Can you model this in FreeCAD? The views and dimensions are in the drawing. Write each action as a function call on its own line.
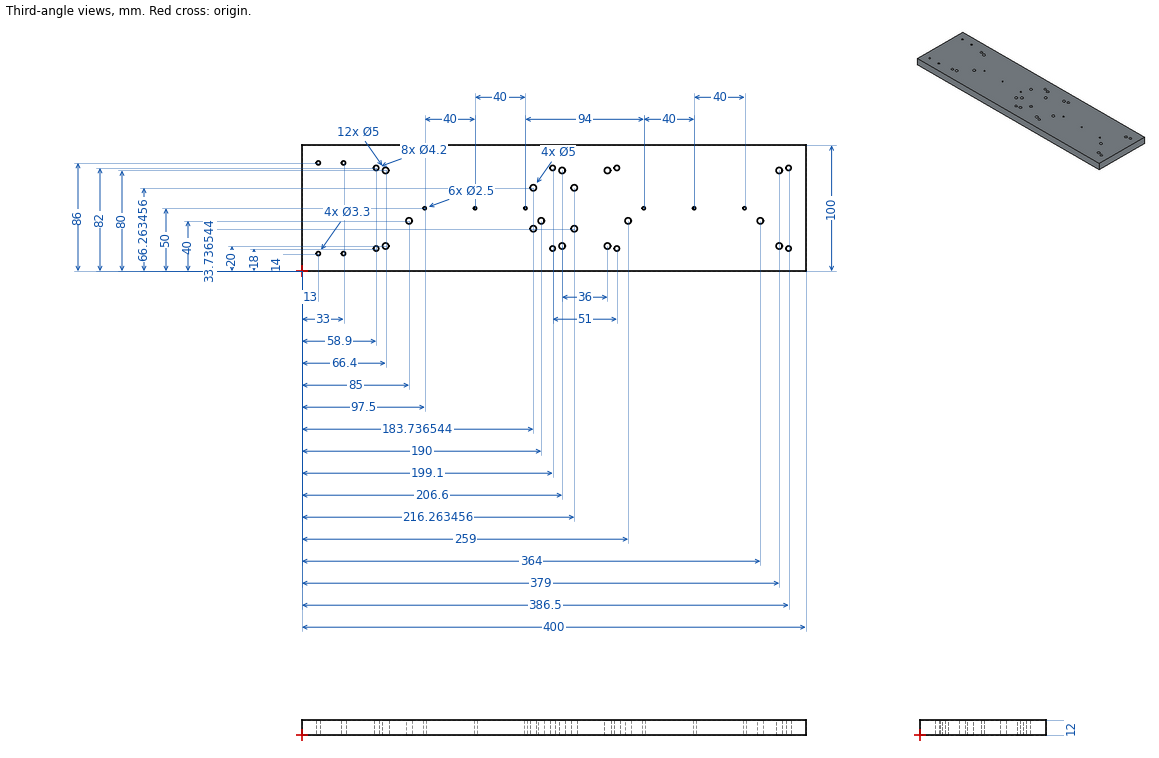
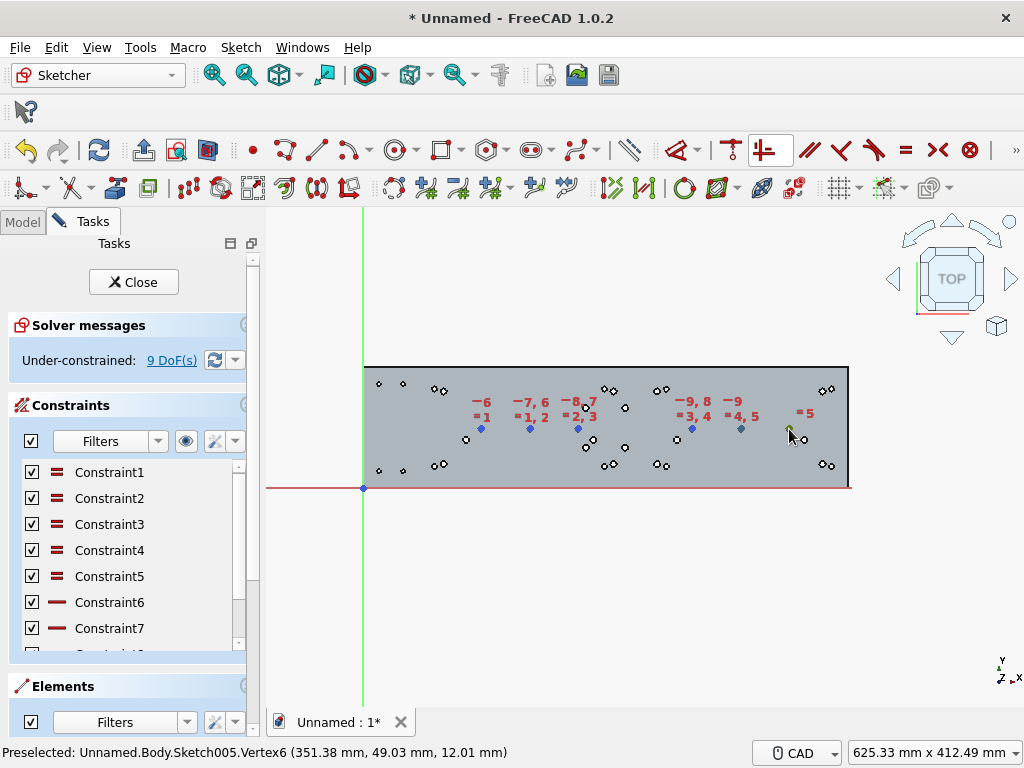
key(h)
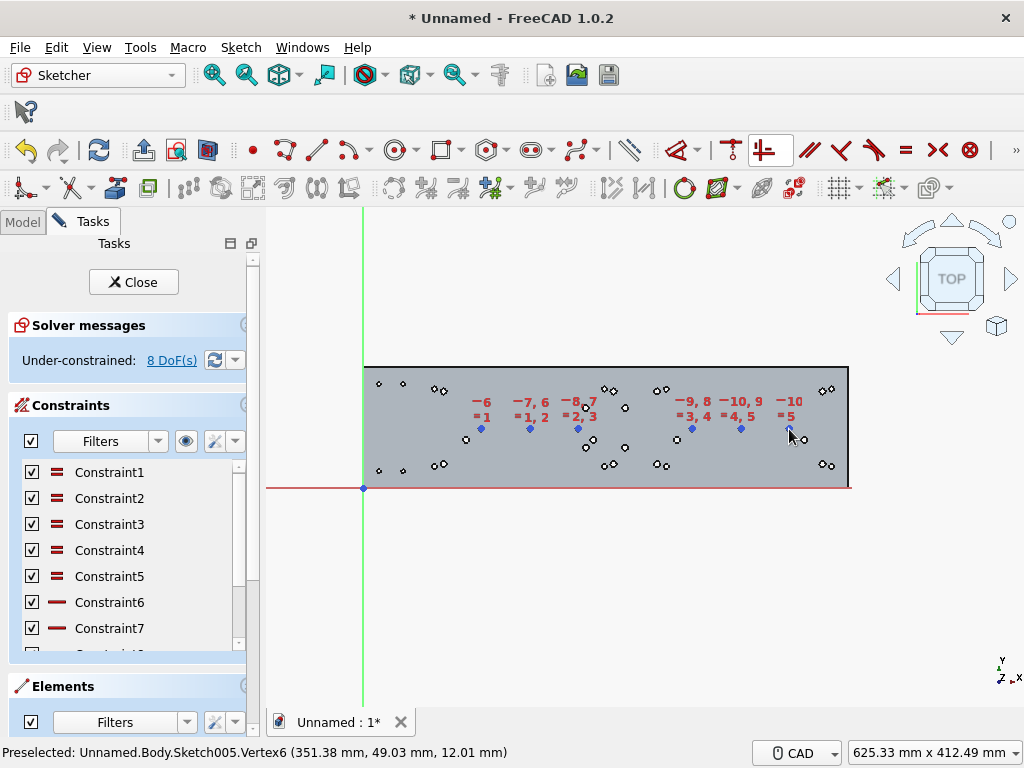
click(676, 150)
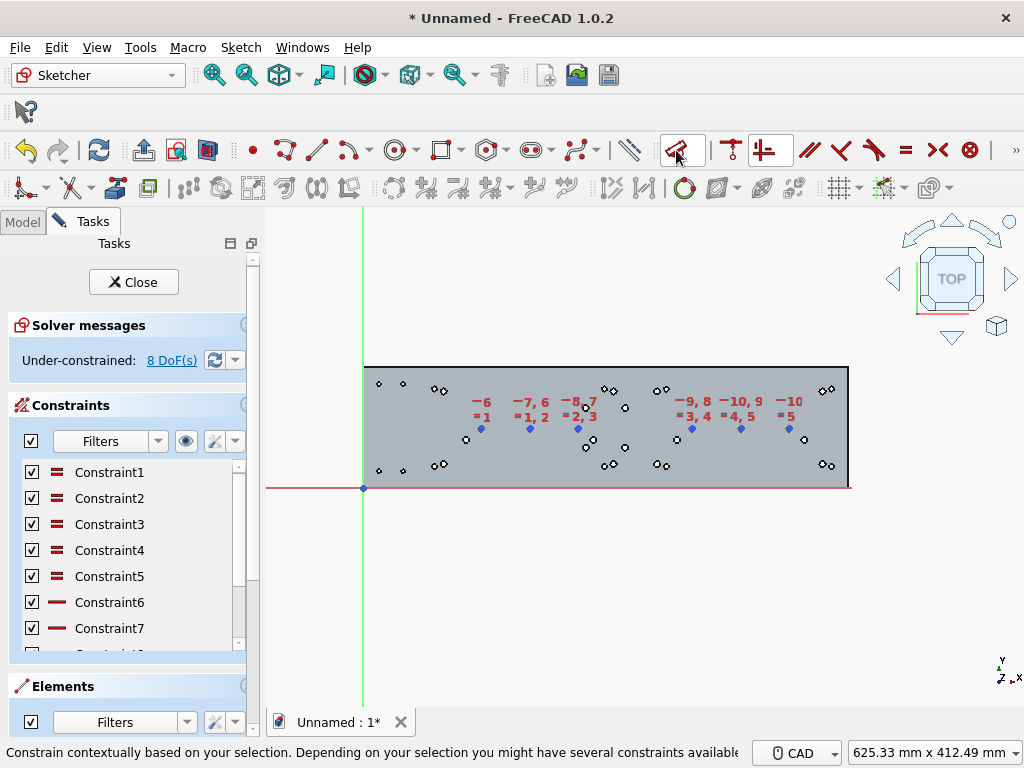
scroll(478, 429, up, 13)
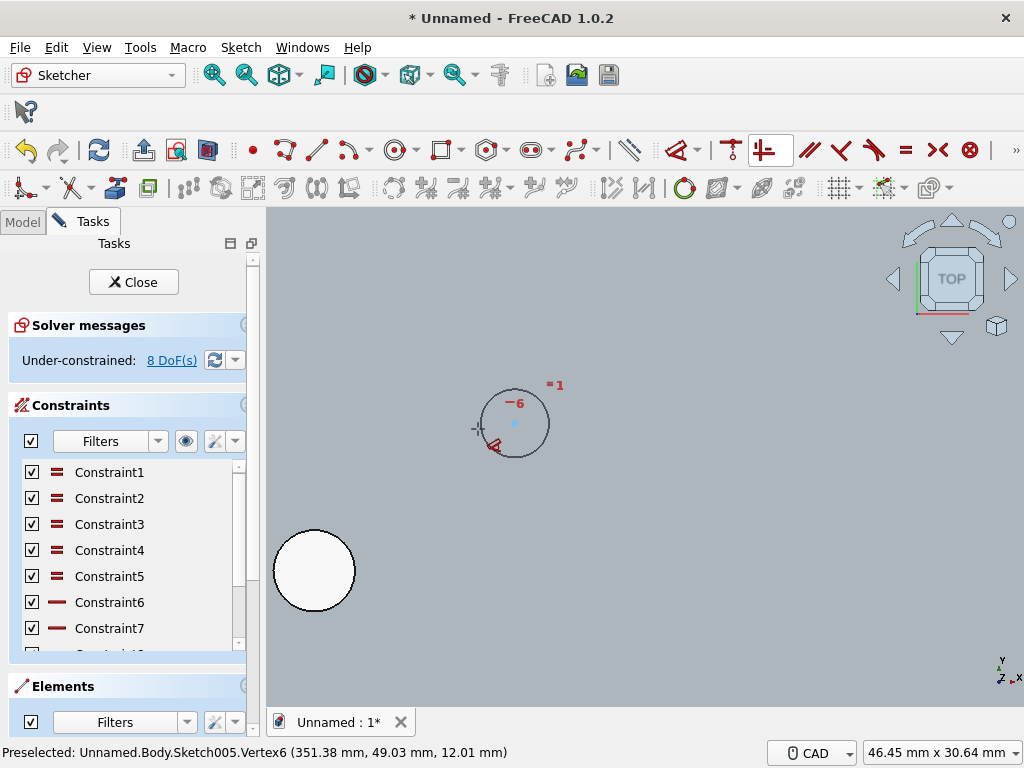
click(481, 422)
click(449, 421)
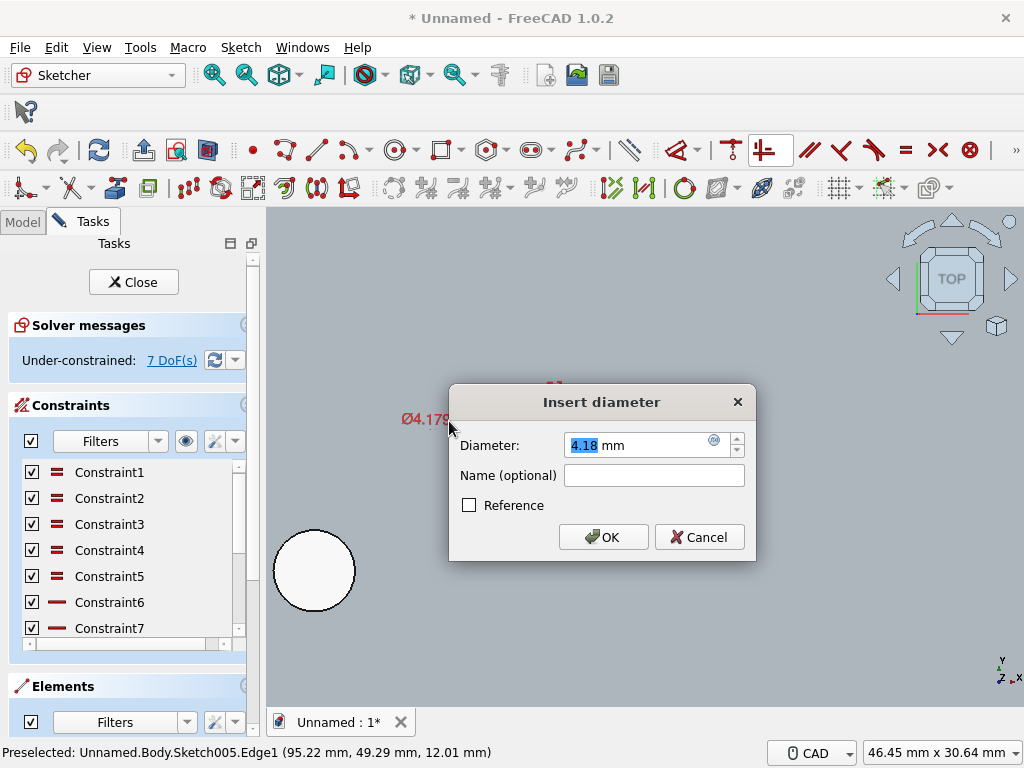
text(2.5)
key(Return)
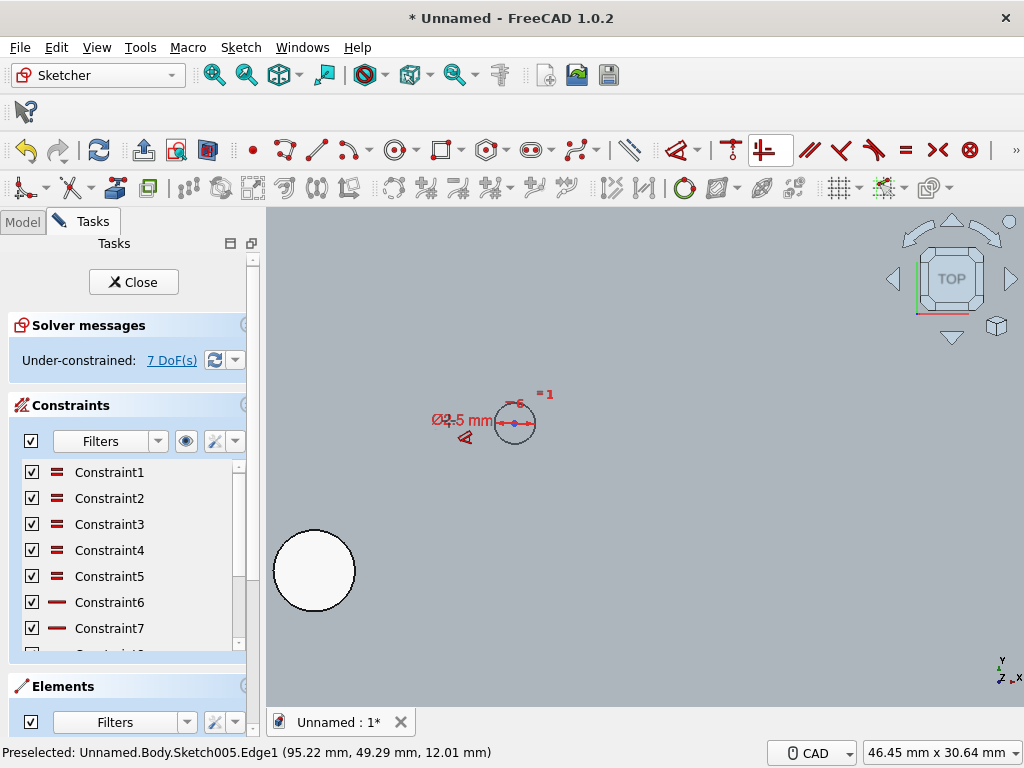
scroll(478, 429, down, 13)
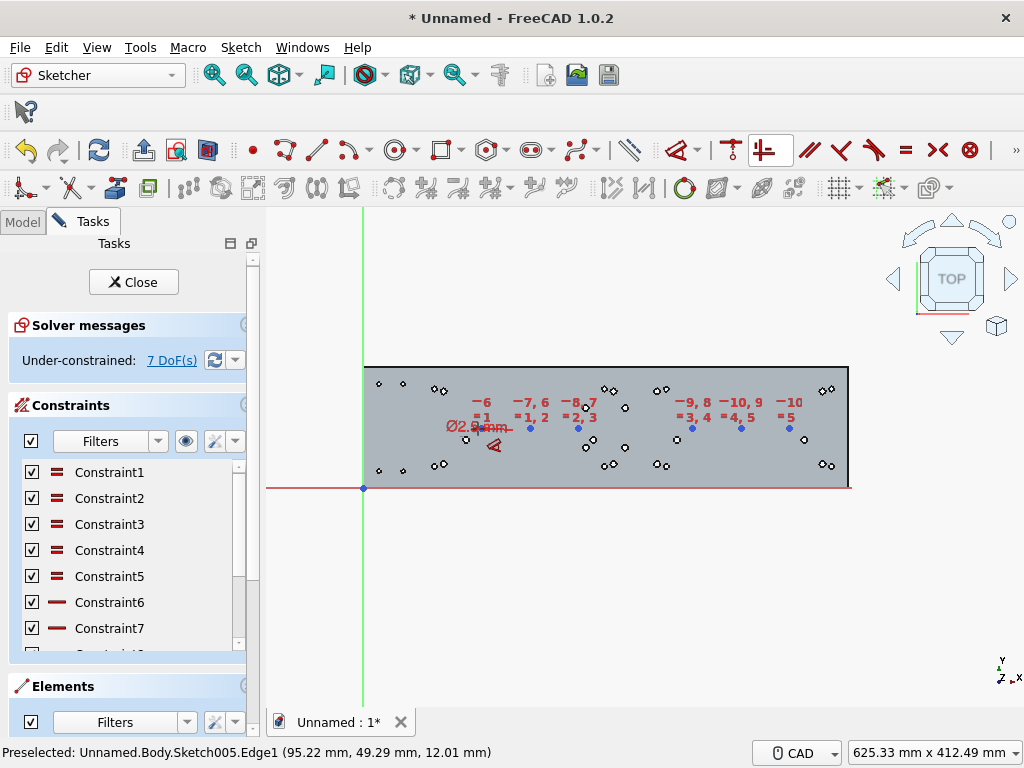
click(481, 429)
click(329, 459)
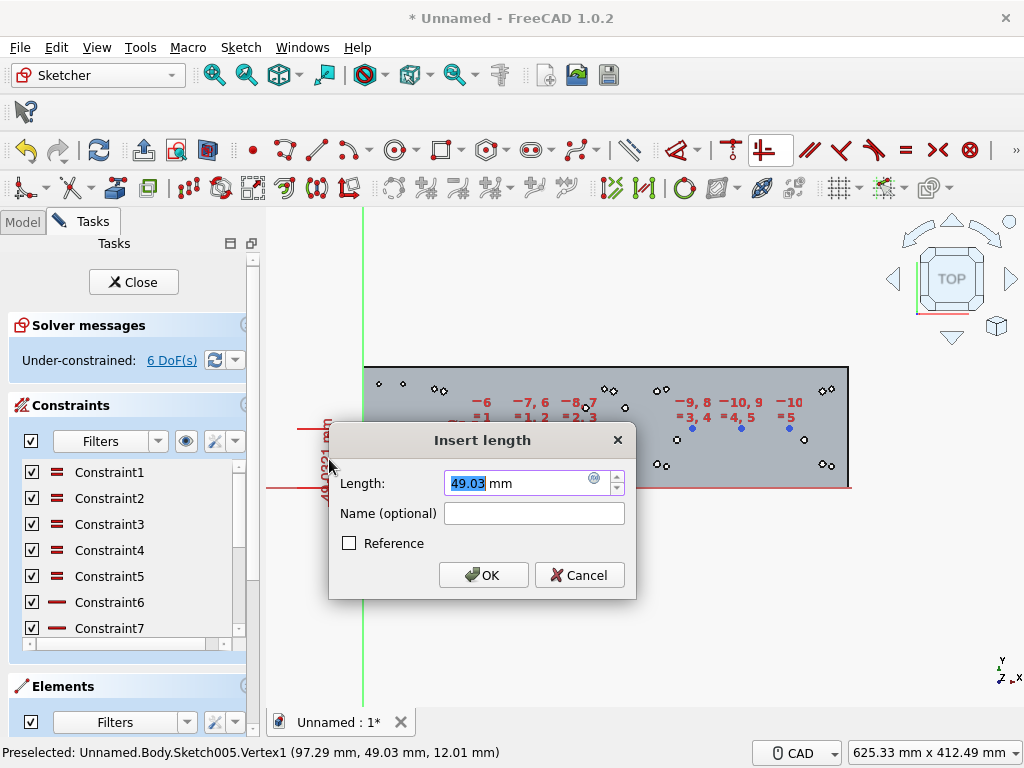
text(50)
key(Return)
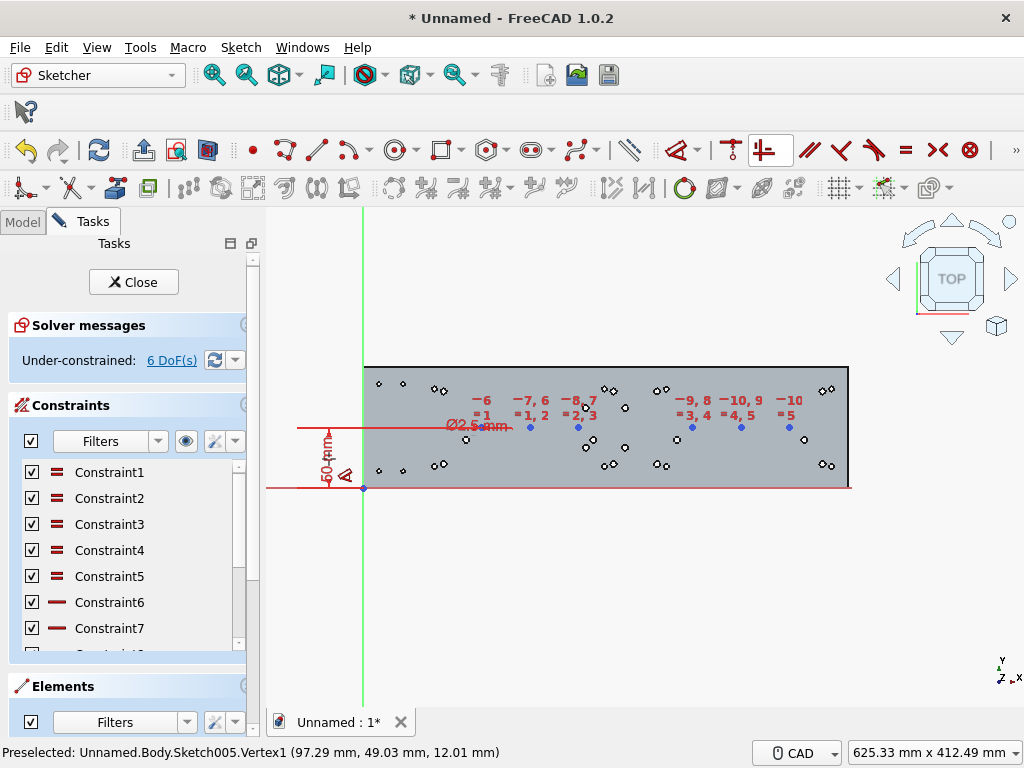
click(481, 428)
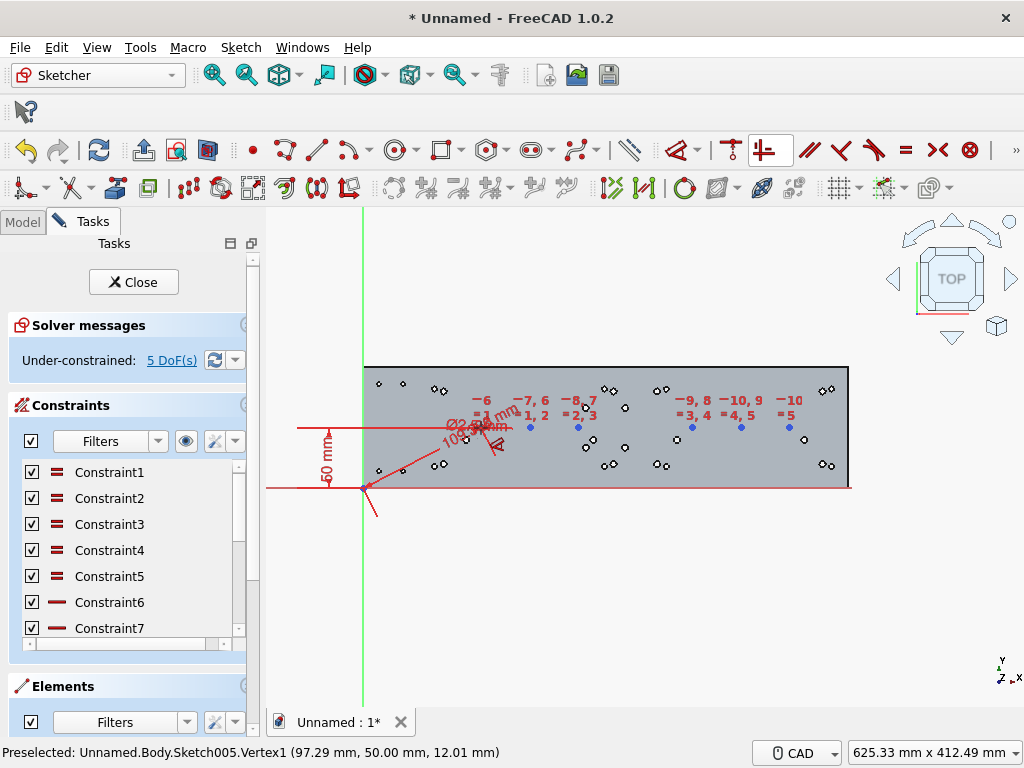
click(530, 428)
click(506, 394)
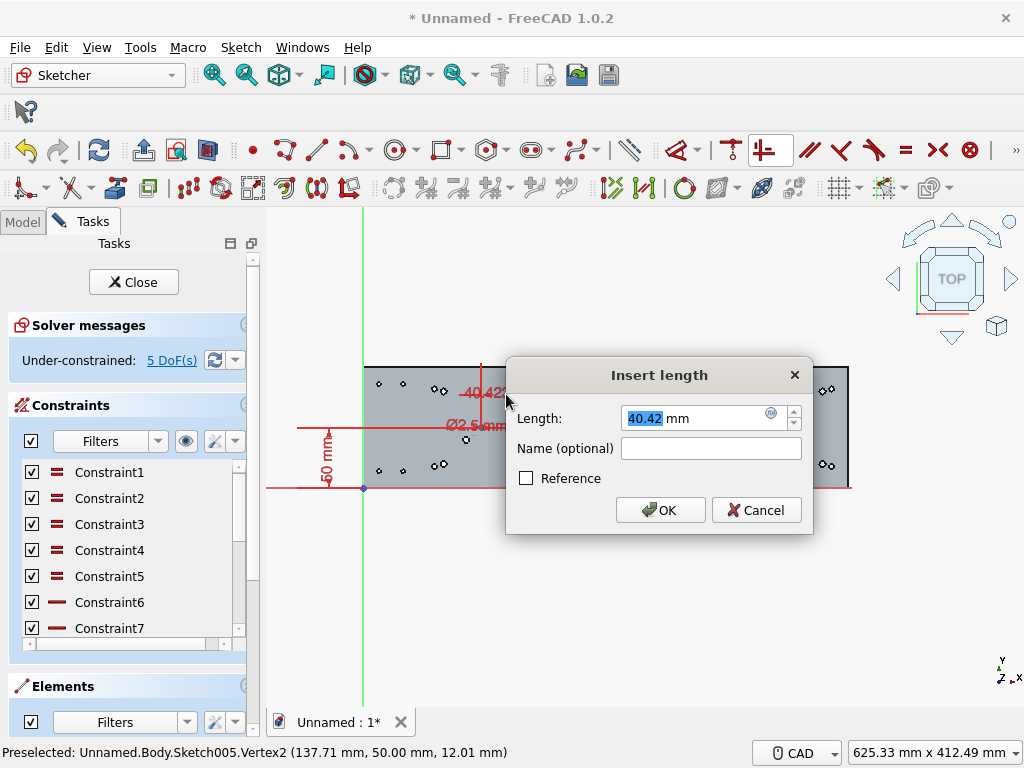
text(40)
key(Return)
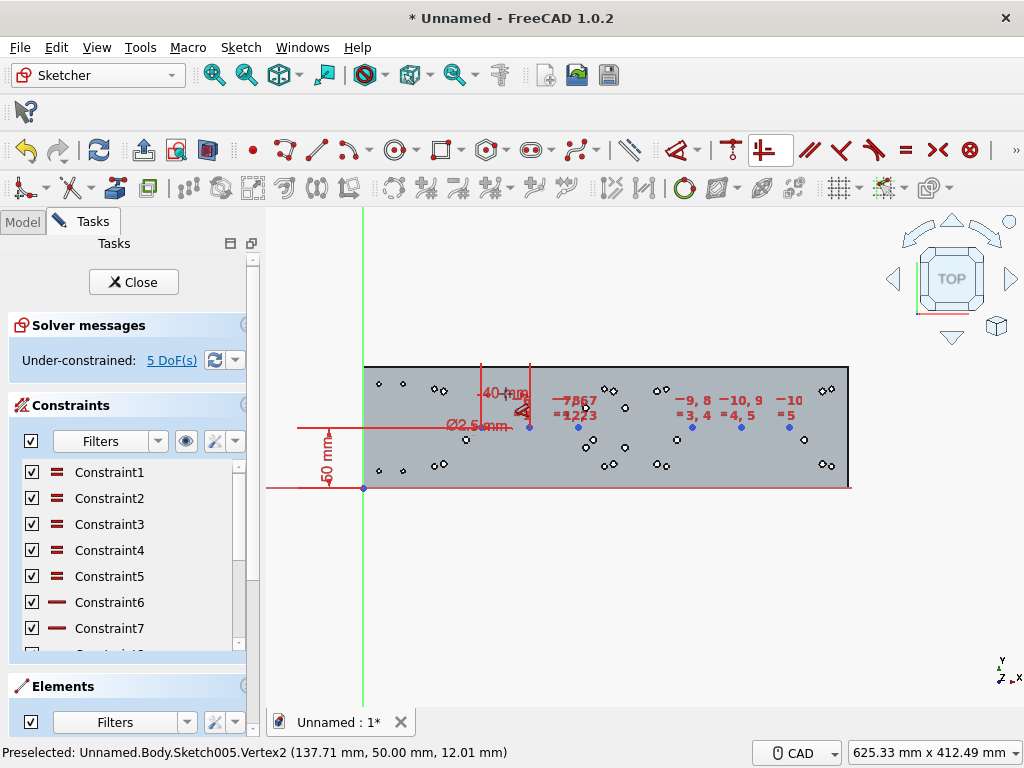
click(530, 428)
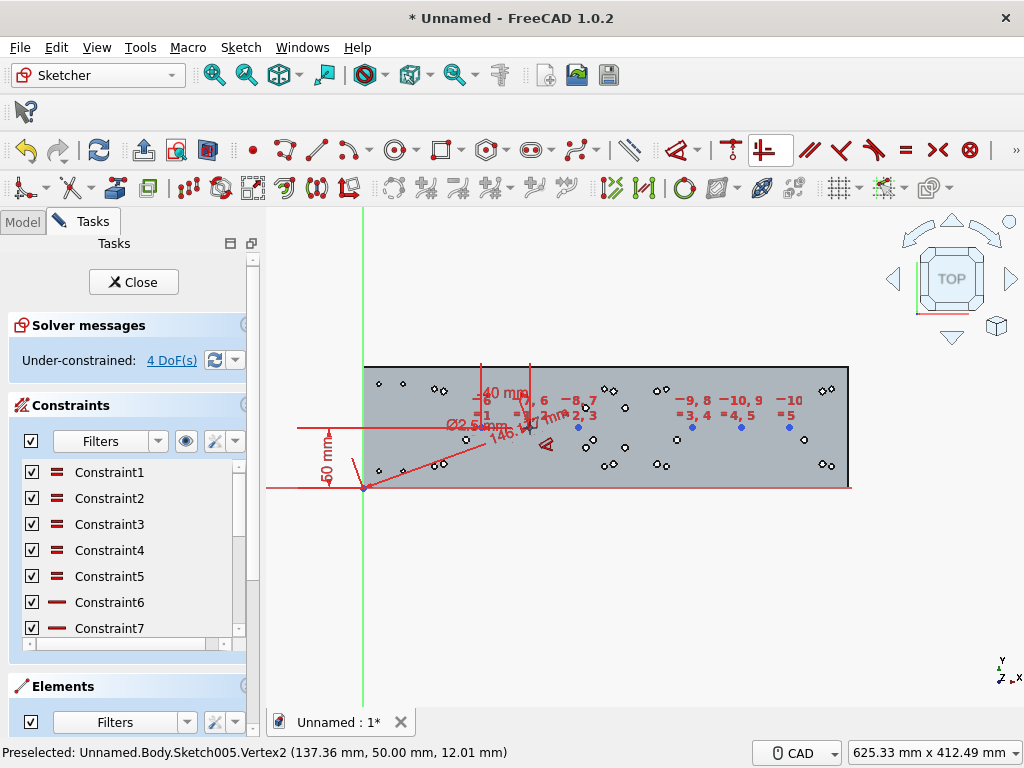
click(578, 428)
click(554, 462)